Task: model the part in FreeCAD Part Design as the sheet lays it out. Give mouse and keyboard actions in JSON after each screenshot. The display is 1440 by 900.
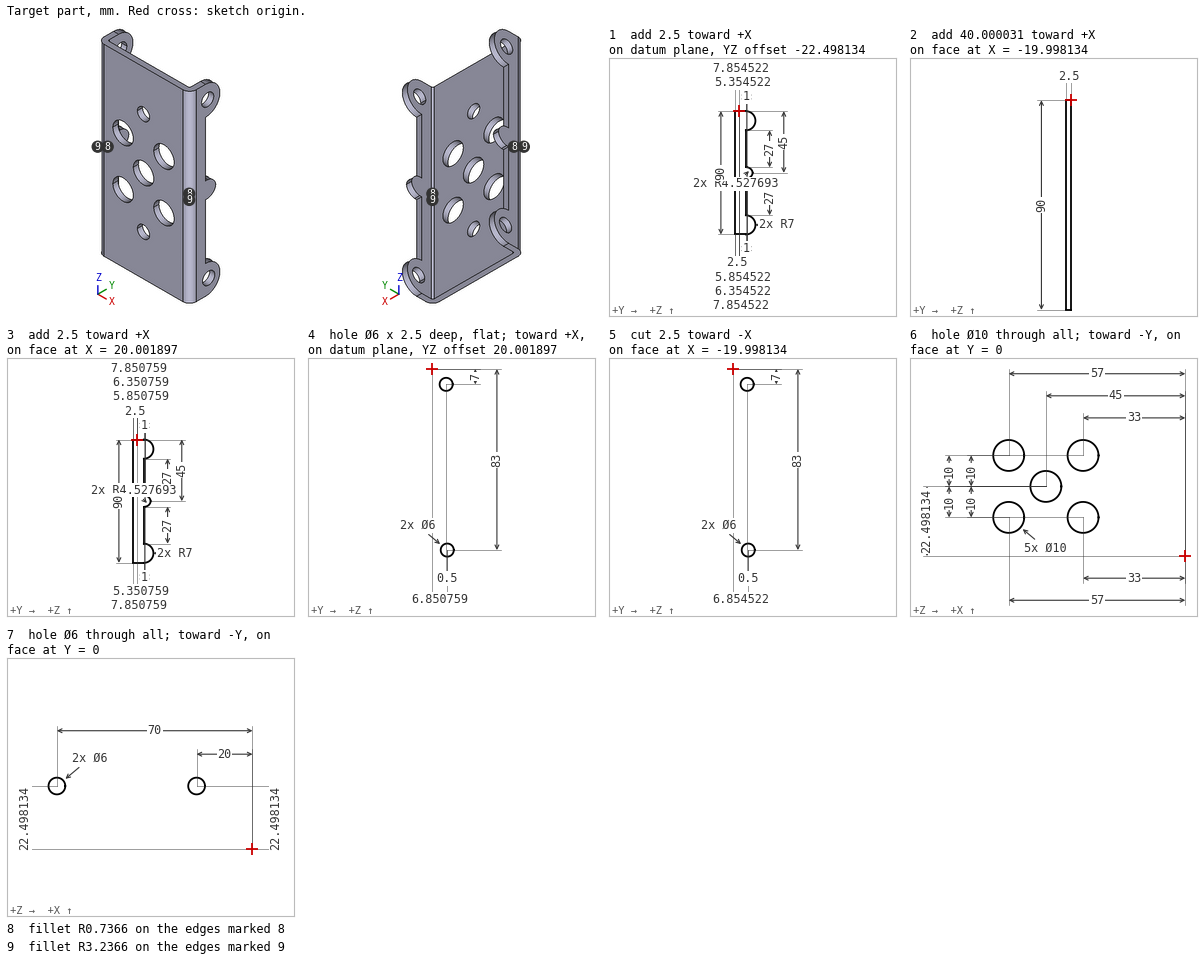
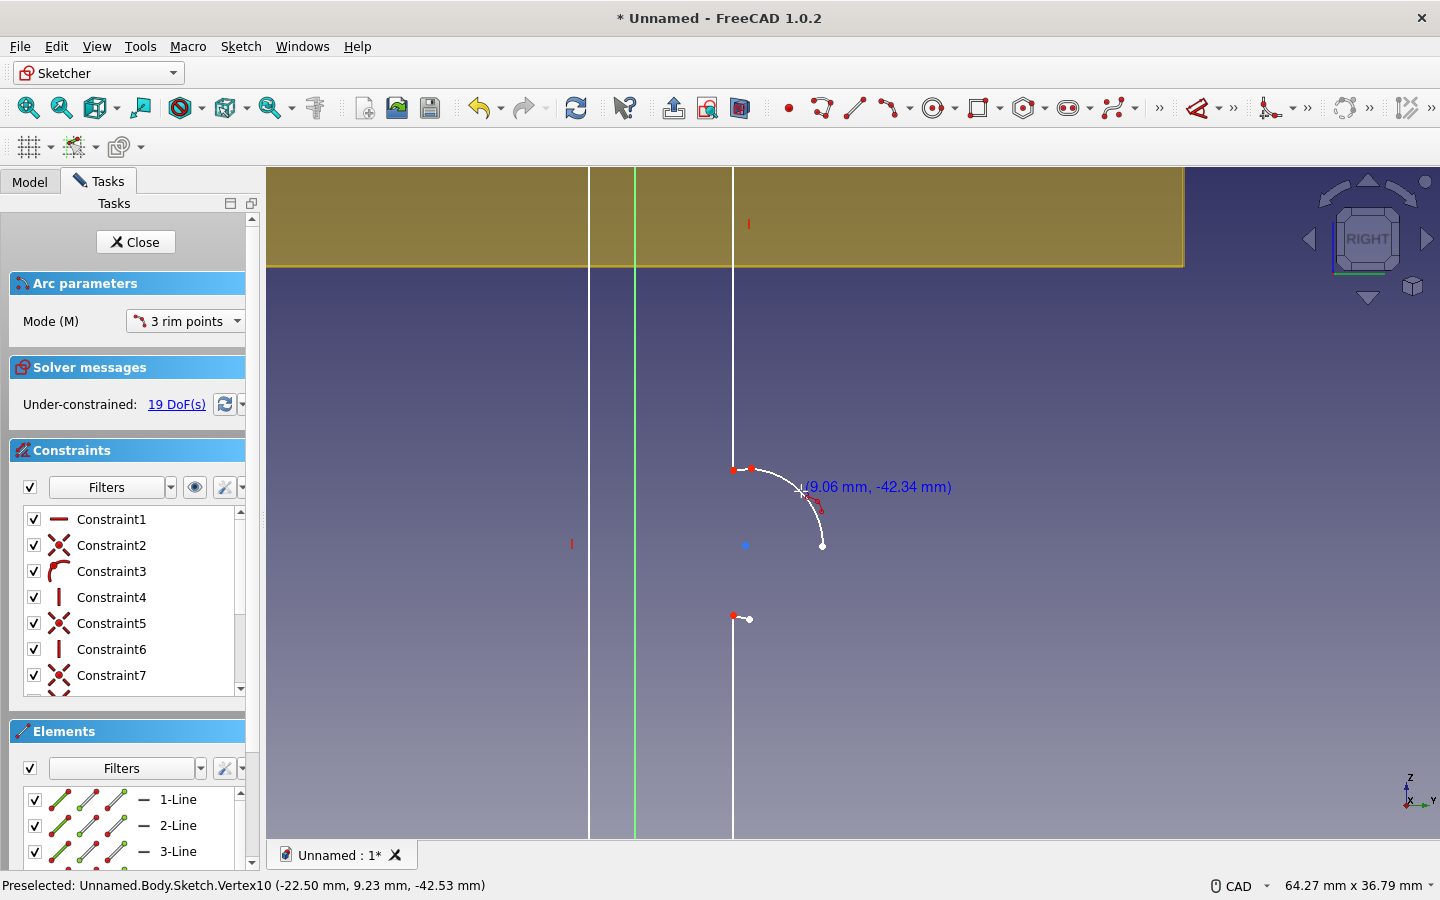
{"action": "scroll", "coordinate": [804, 491], "scroll_direction": "down", "scroll_amount": 7}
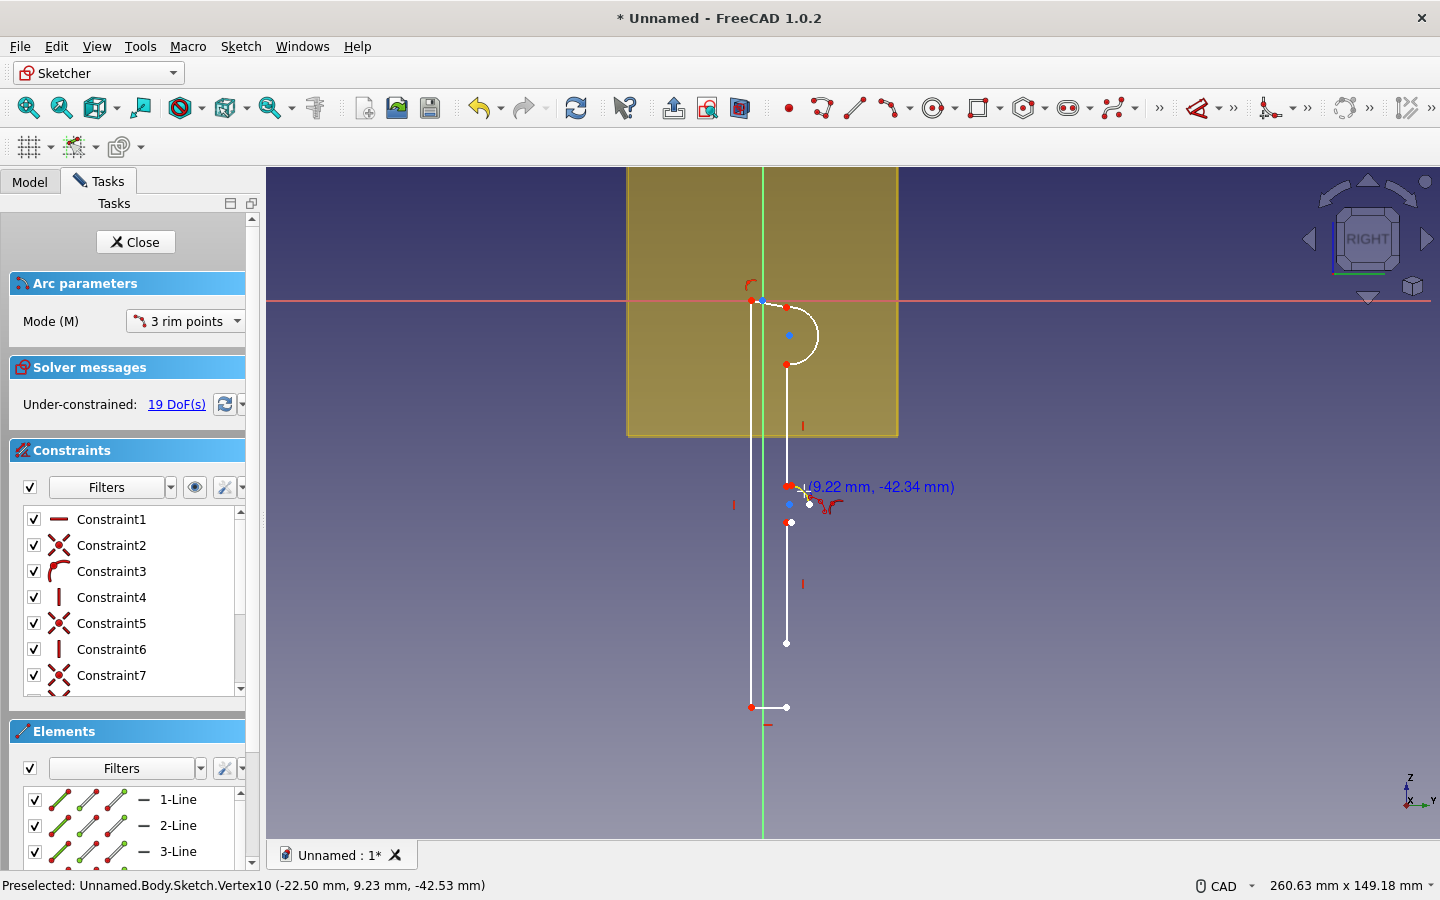
{"action": "left_click", "coordinate": [809, 505]}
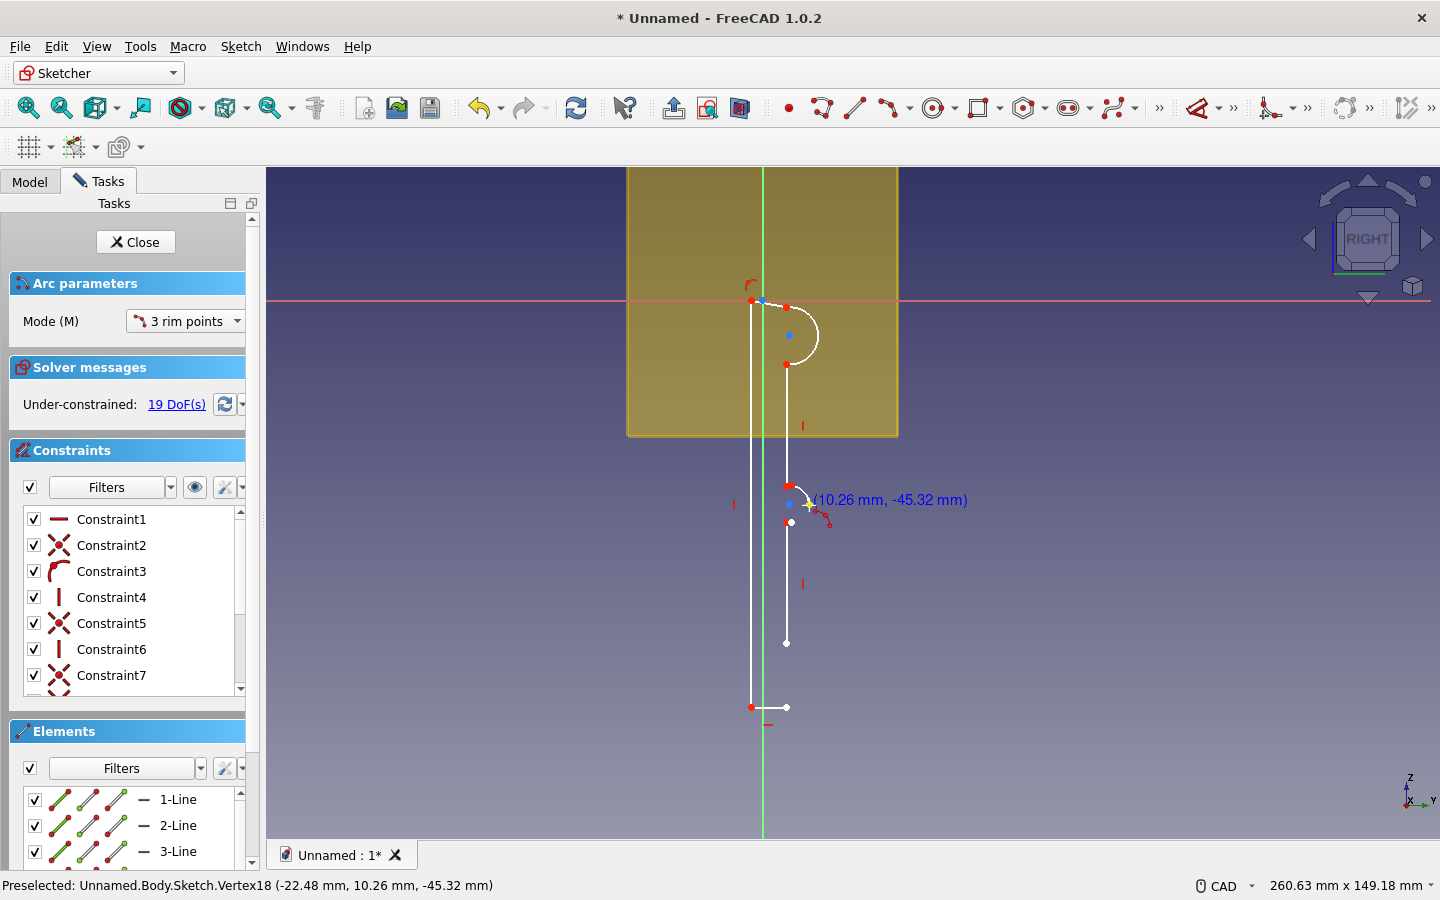
{"action": "scroll", "coordinate": [791, 522], "scroll_direction": "up", "scroll_amount": 10}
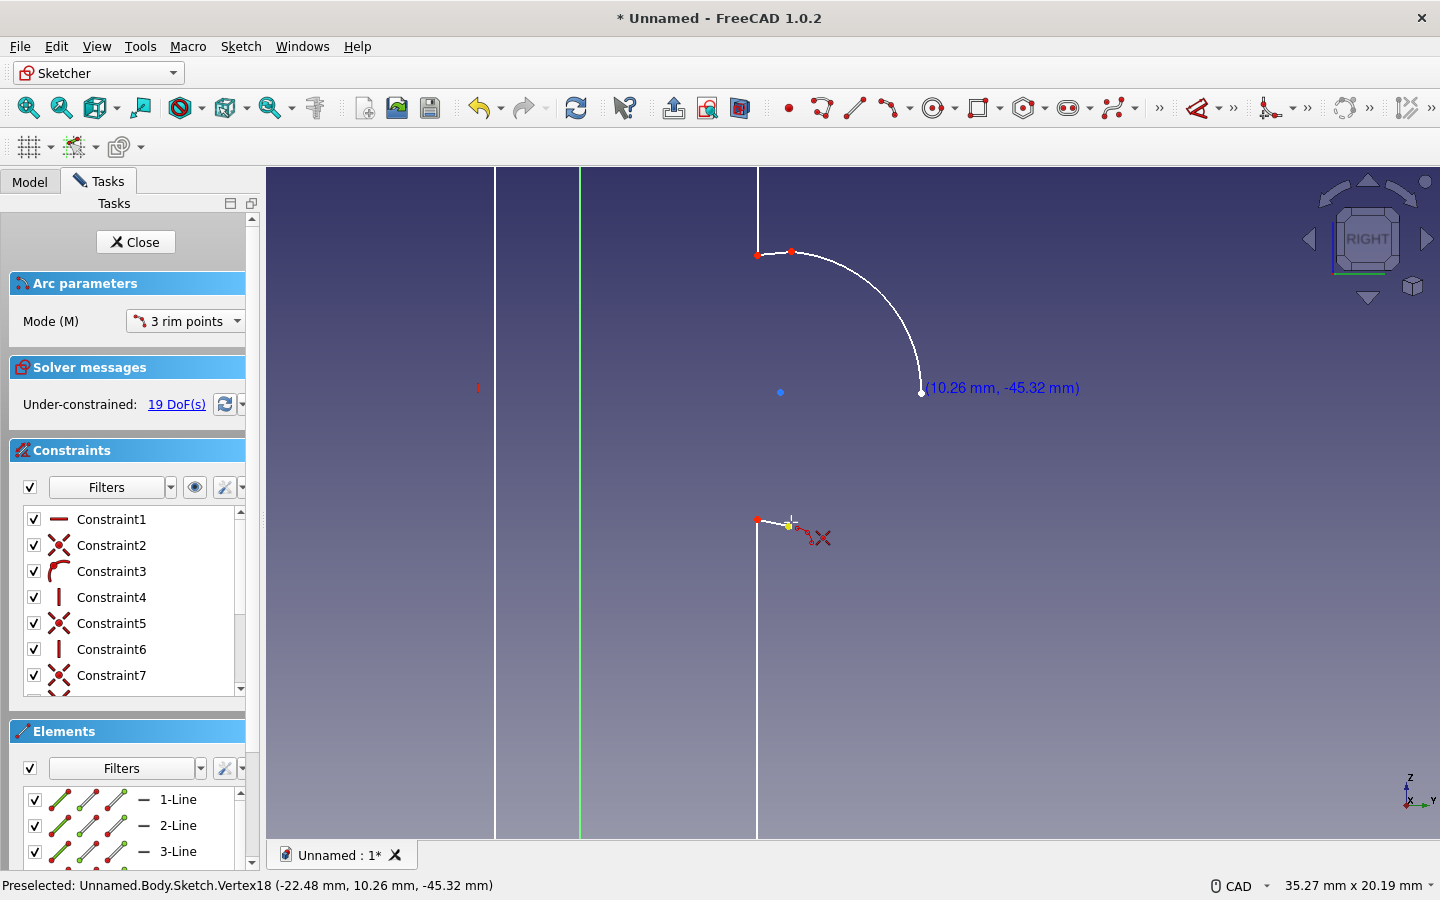
{"action": "left_click", "coordinate": [788, 526]}
{"action": "left_click", "coordinate": [881, 472]}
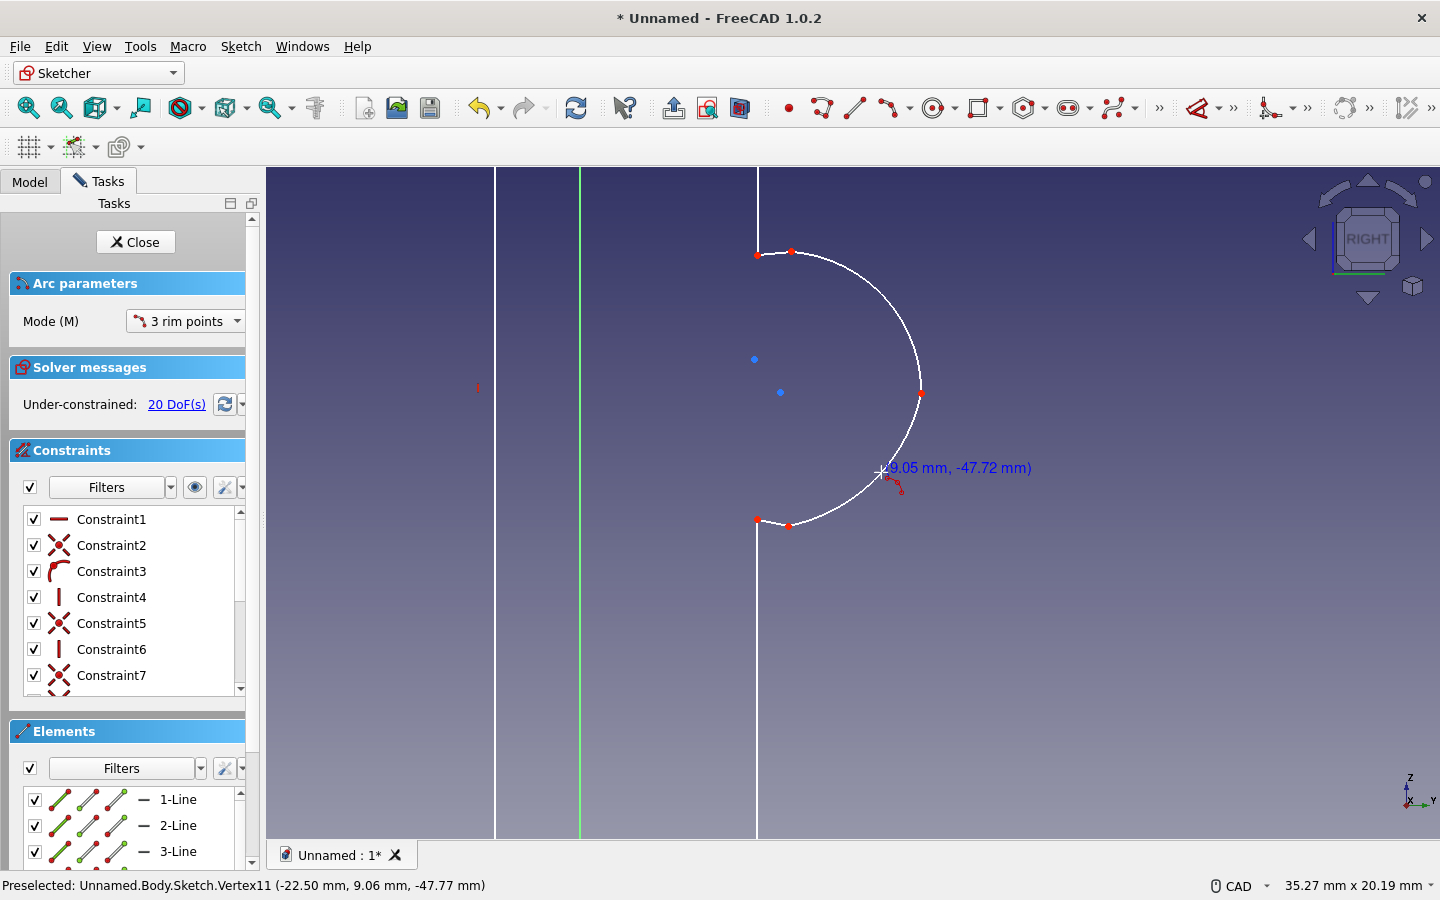
{"action": "scroll", "coordinate": [791, 522], "scroll_direction": "down", "scroll_amount": 10}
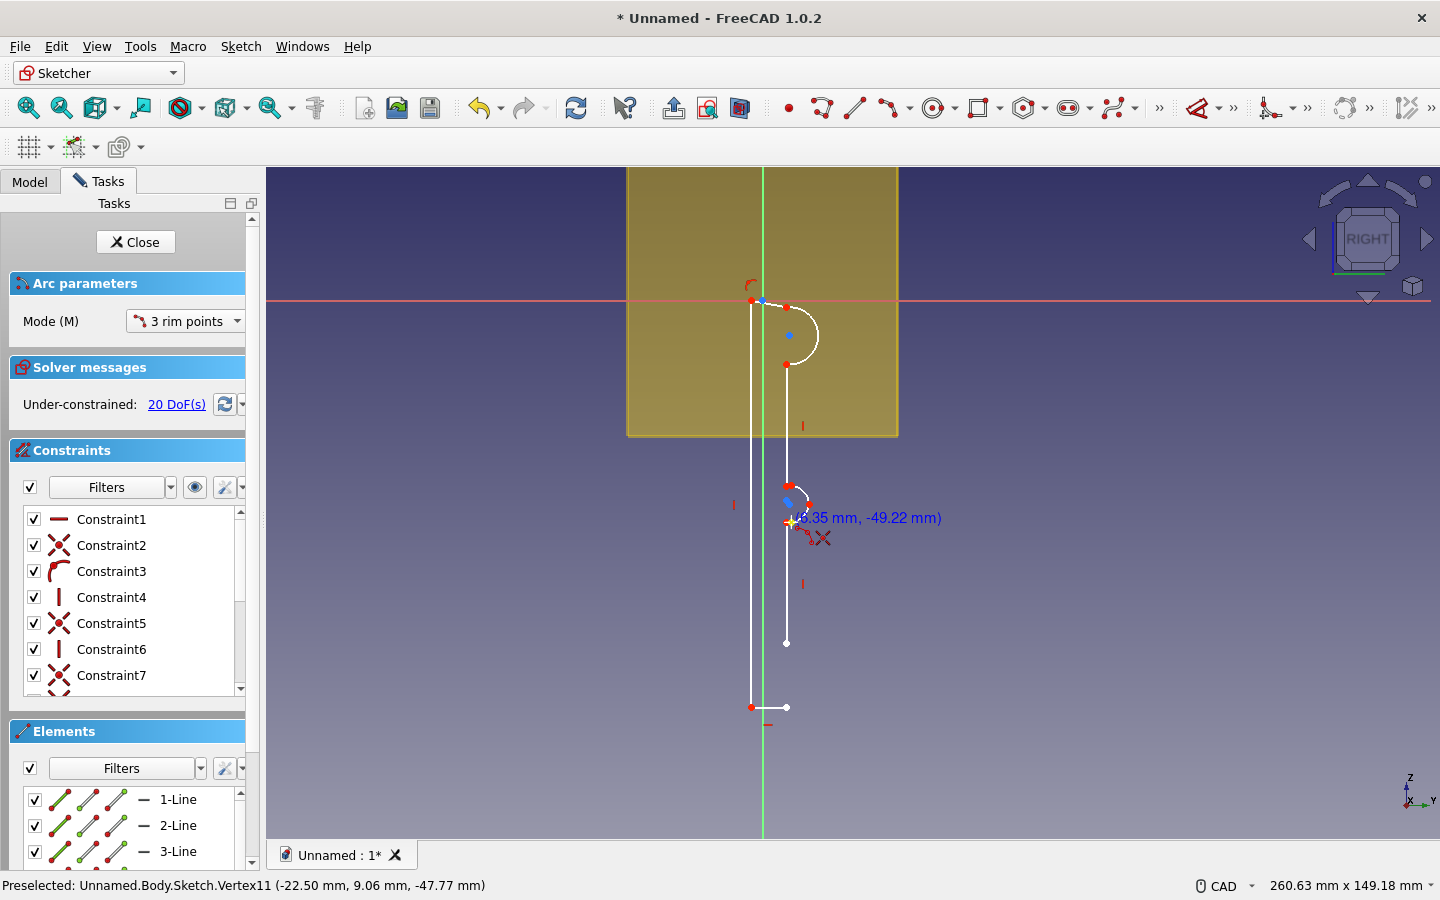
{"action": "left_click", "coordinate": [787, 644]}
{"action": "left_click", "coordinate": [787, 708]}
{"action": "left_click", "coordinate": [818, 675]}
{"action": "key", "text": "Escape"}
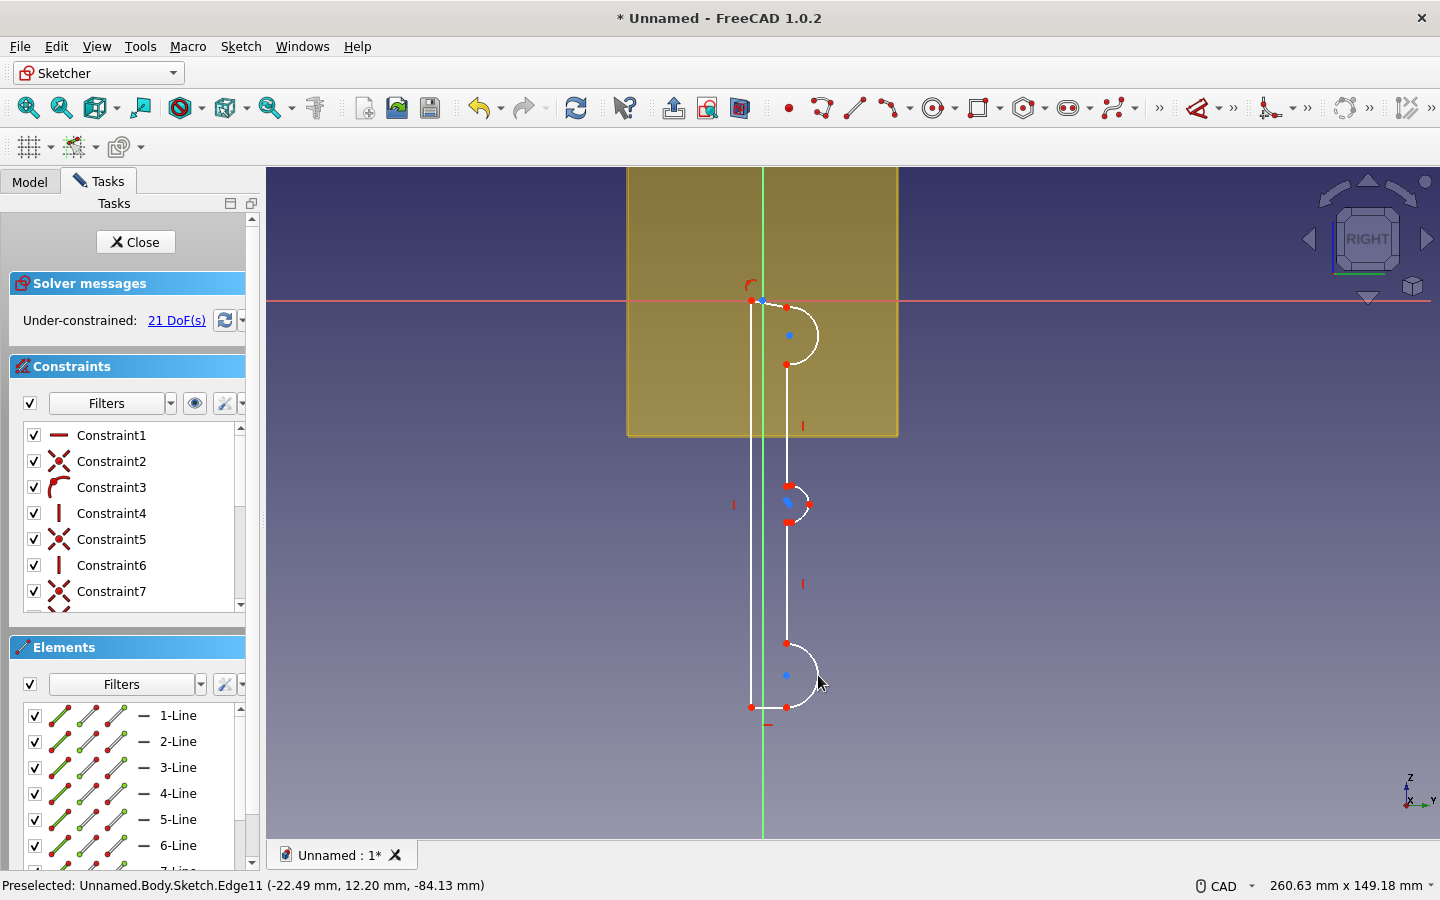
{"action": "scroll", "coordinate": [776, 708], "scroll_direction": "up", "scroll_amount": 2}